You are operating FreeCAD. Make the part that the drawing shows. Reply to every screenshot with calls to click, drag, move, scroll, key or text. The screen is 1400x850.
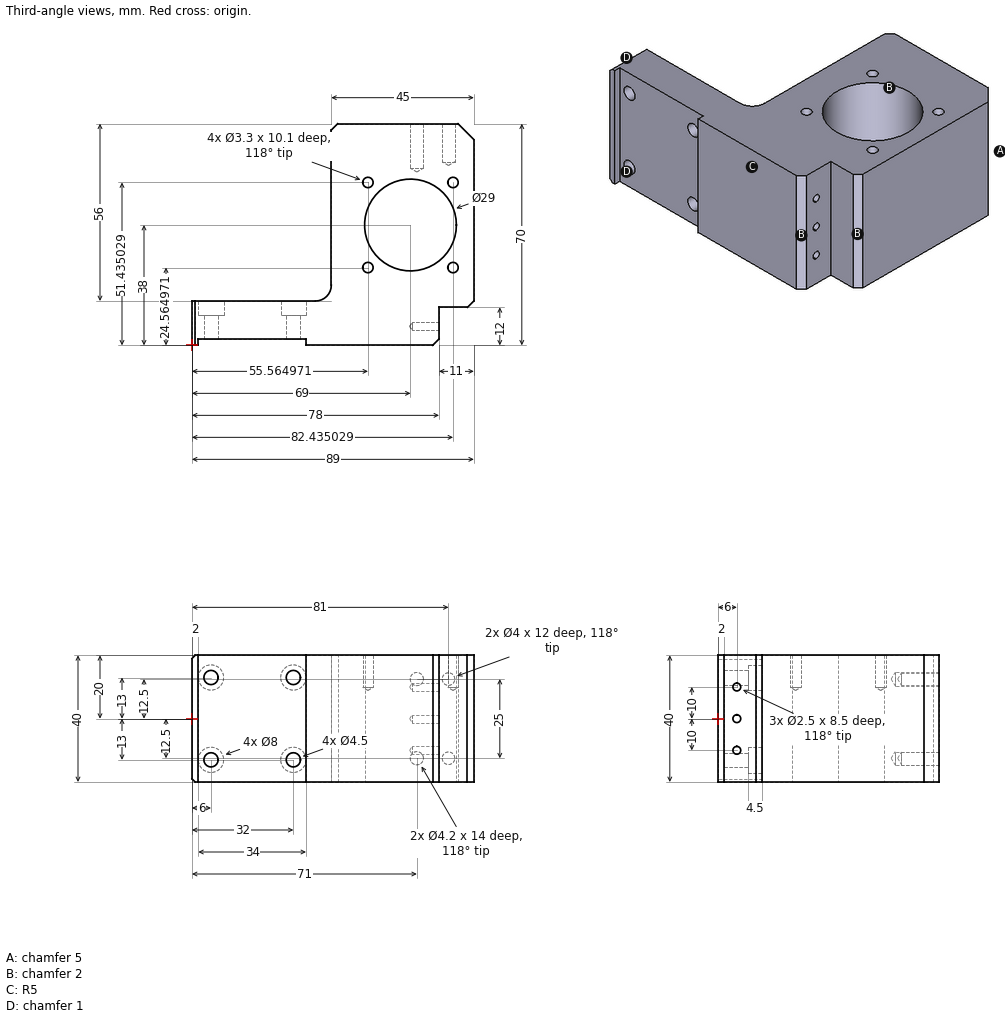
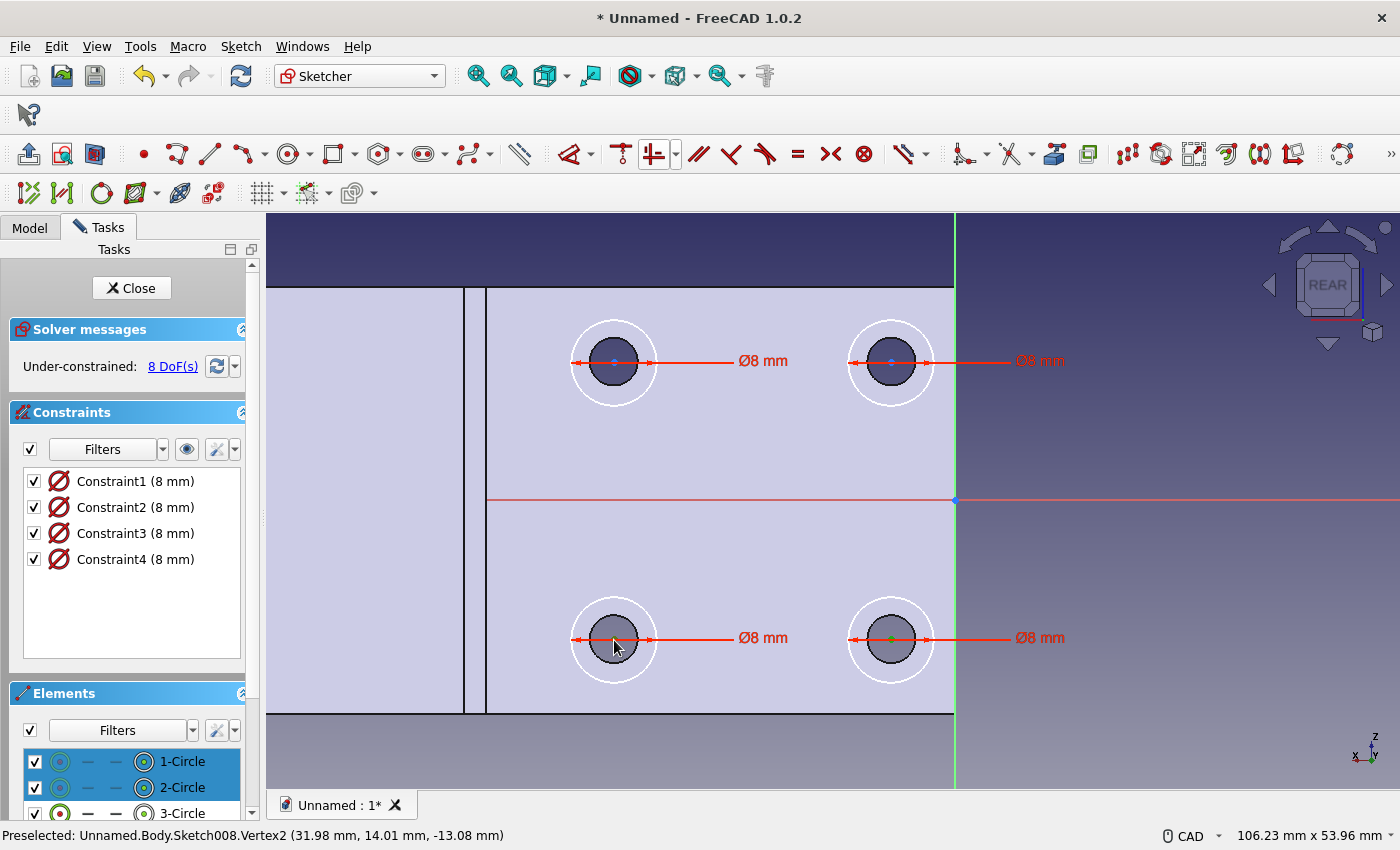
key(h)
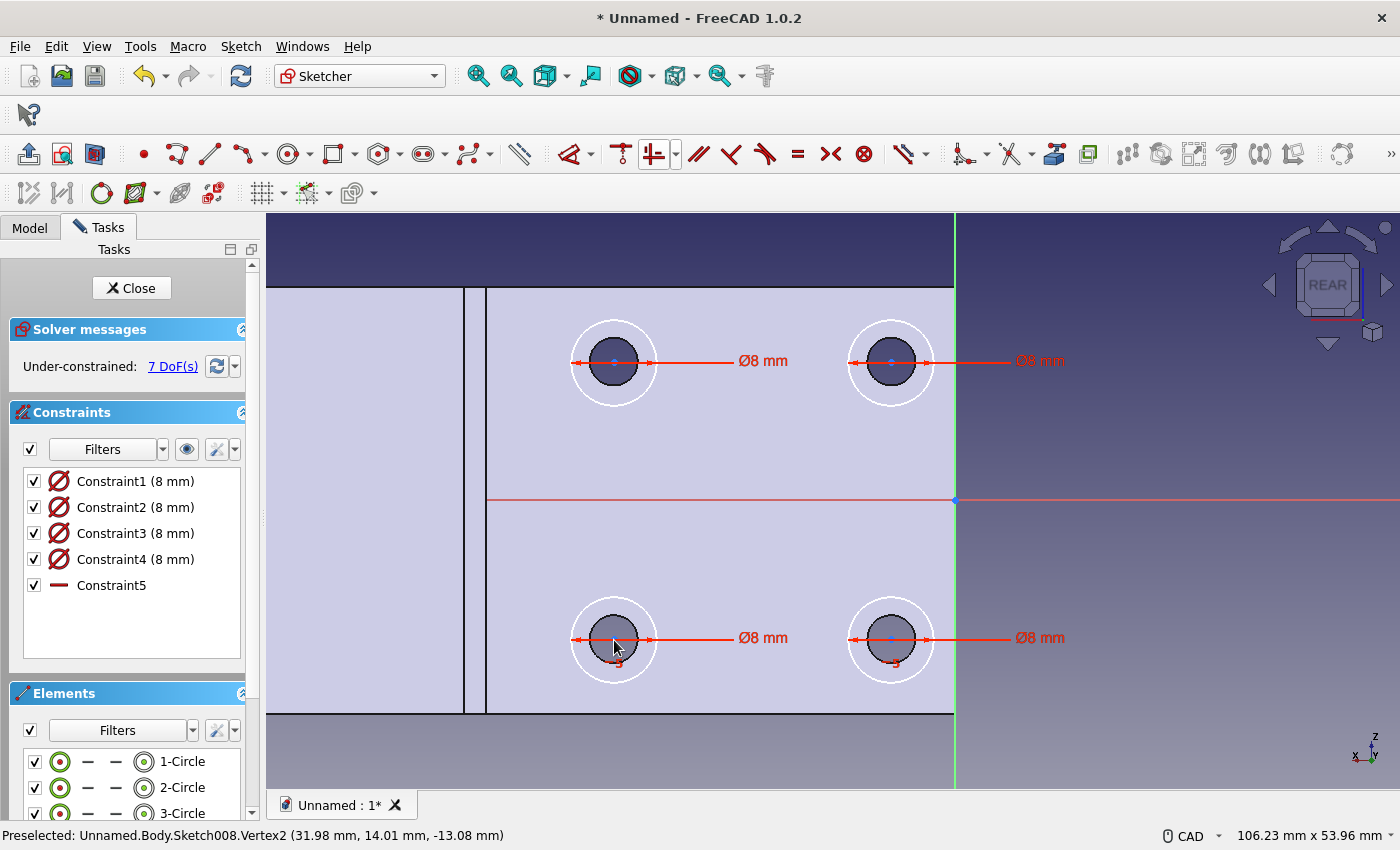
click(614, 640)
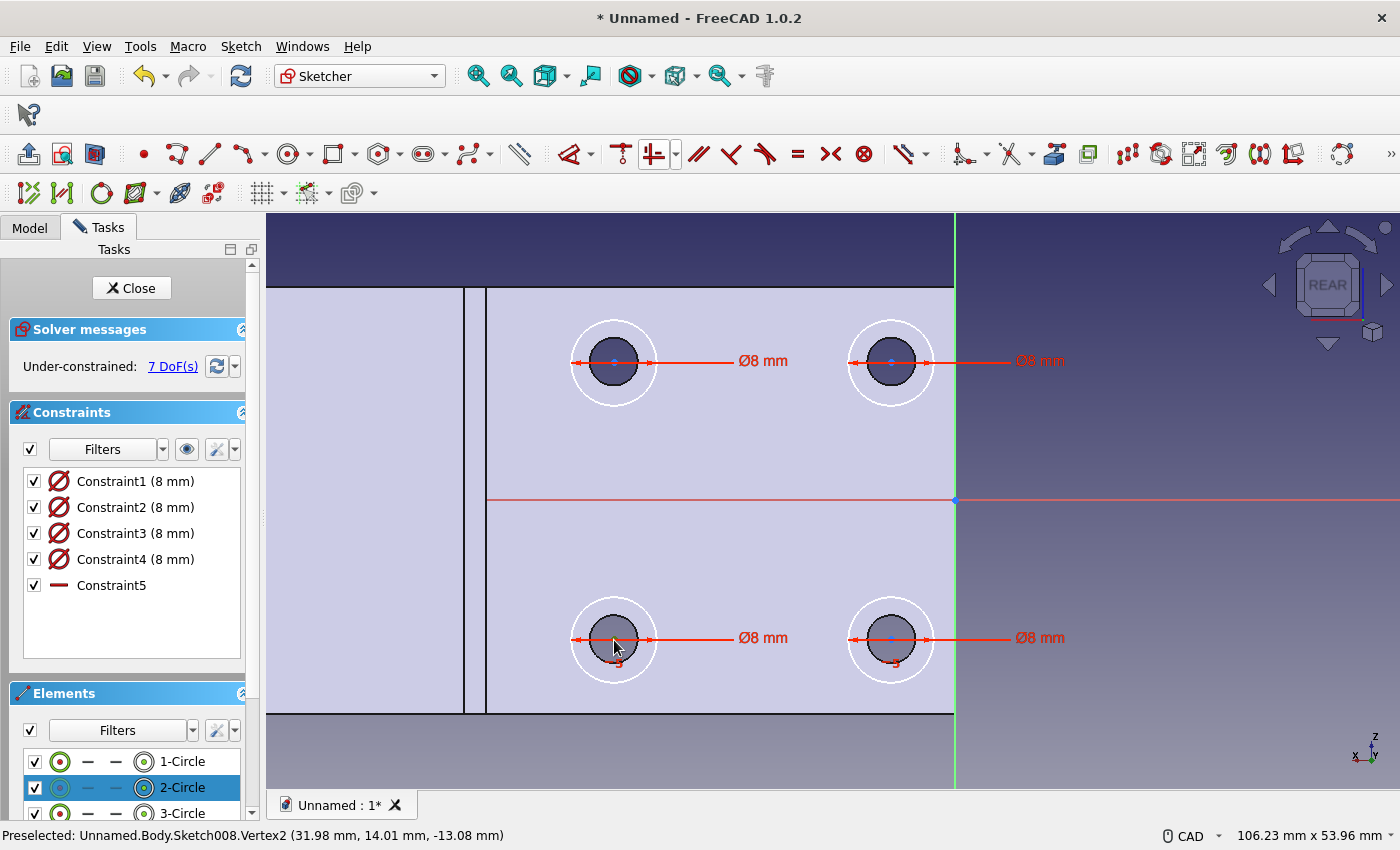
click(614, 363)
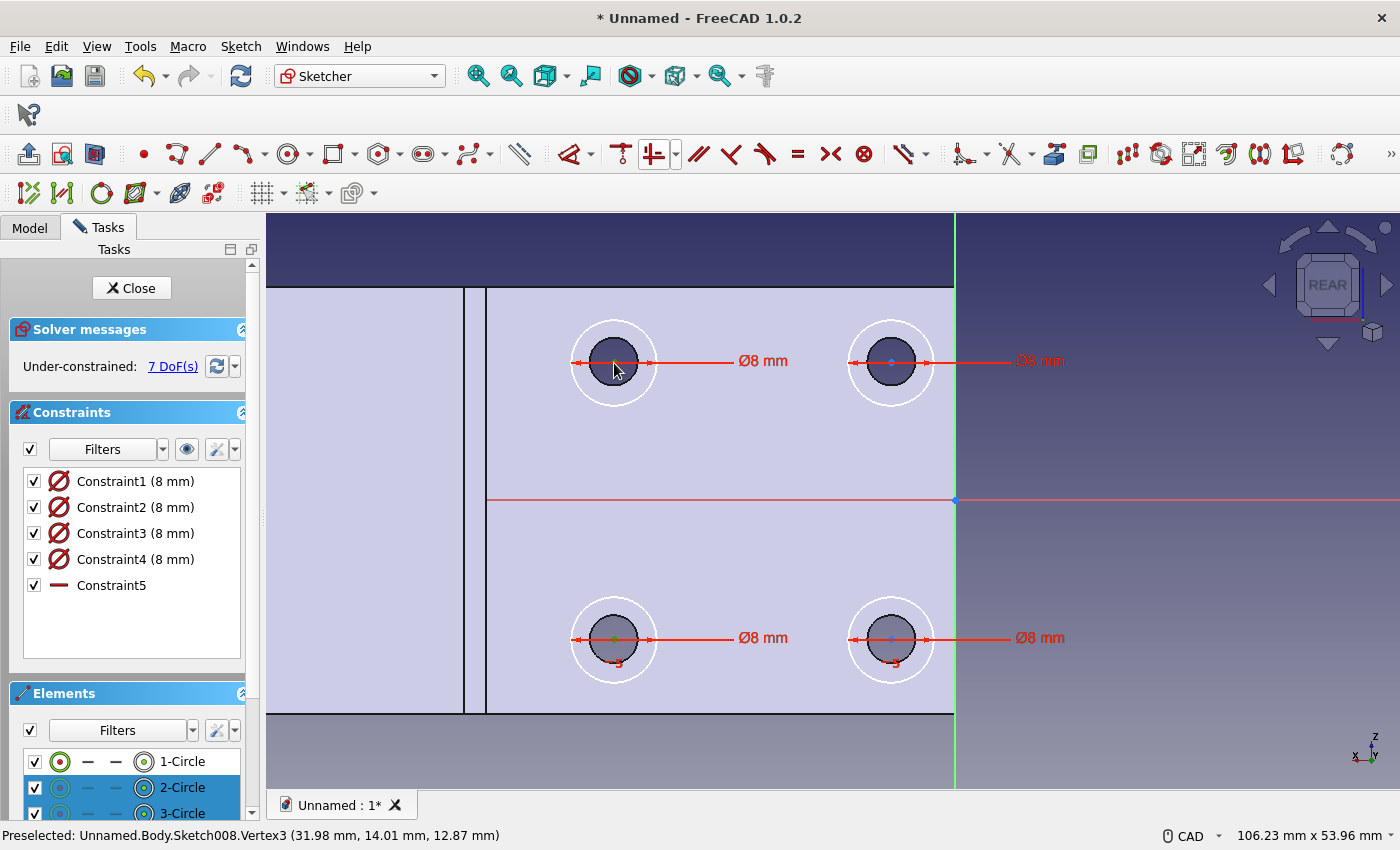
key(v)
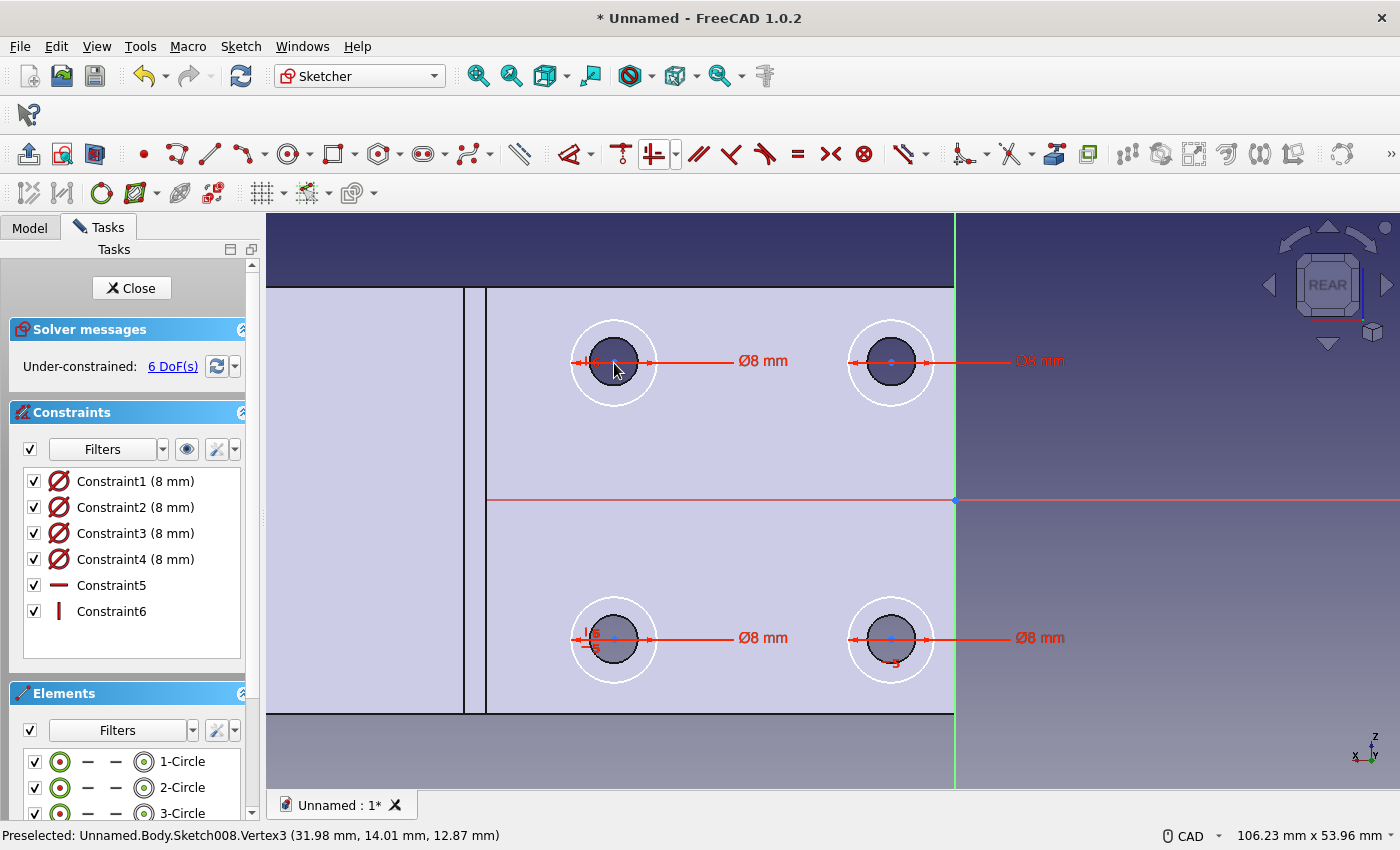
click(891, 640)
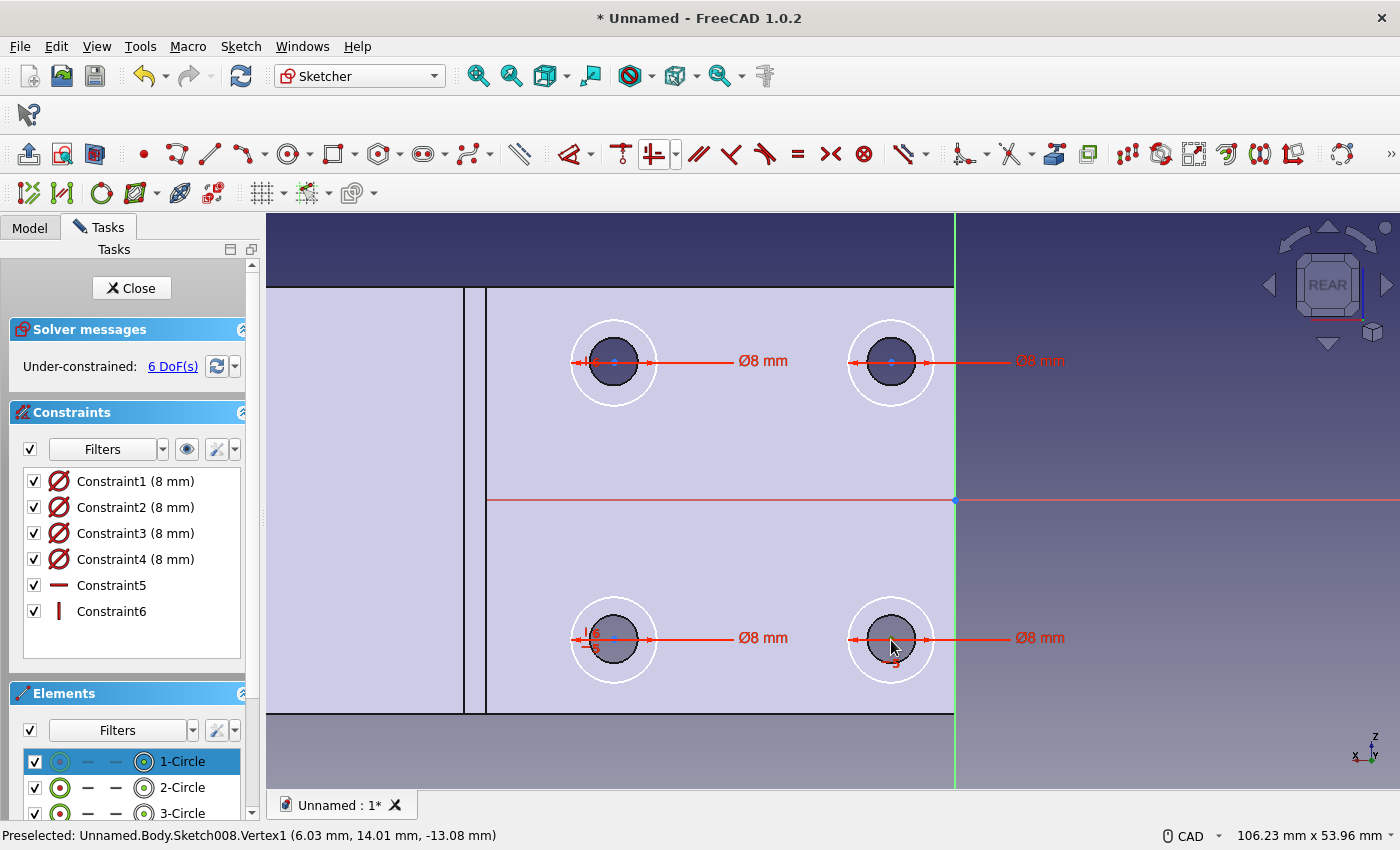
click(891, 363)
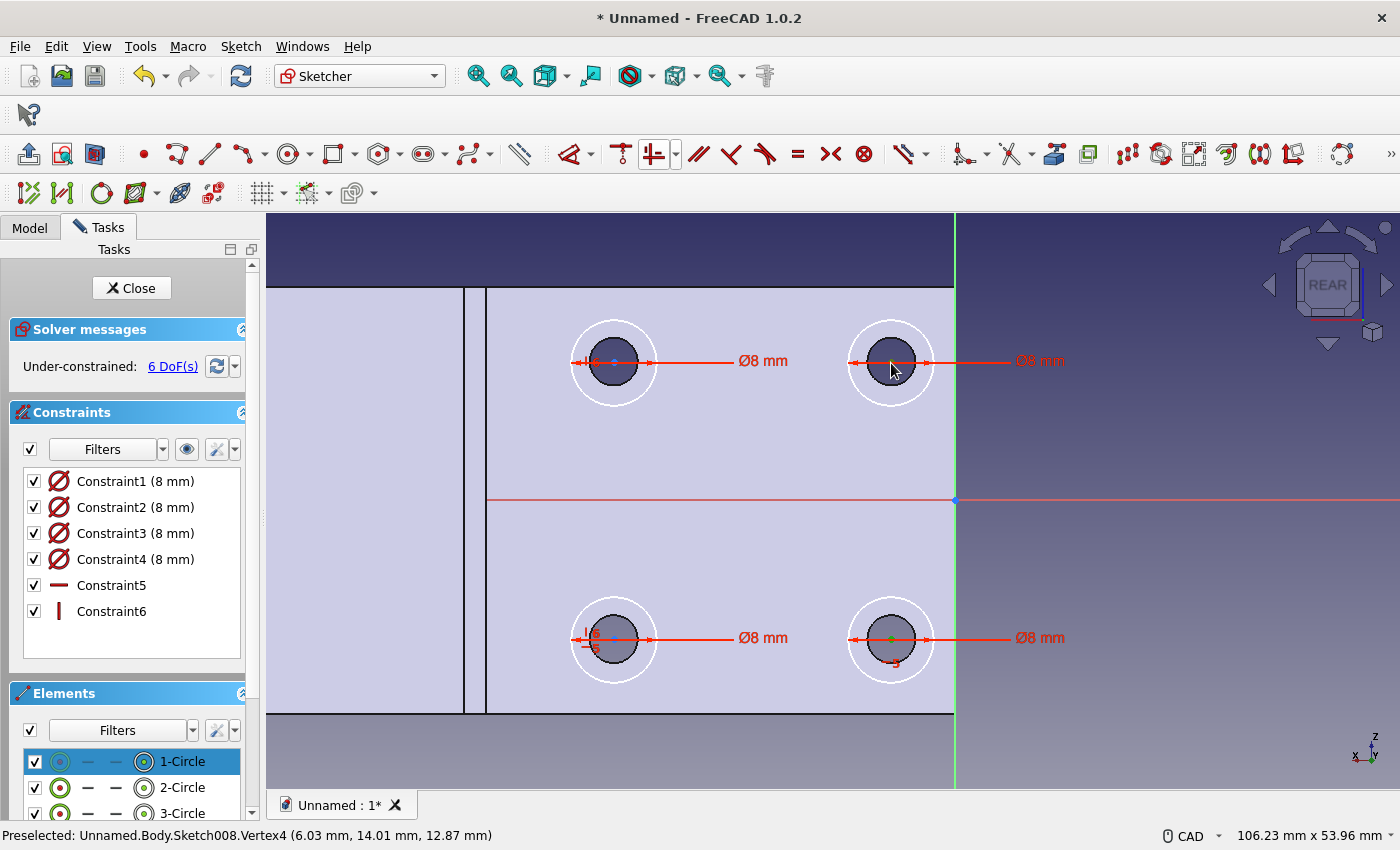
click(676, 154)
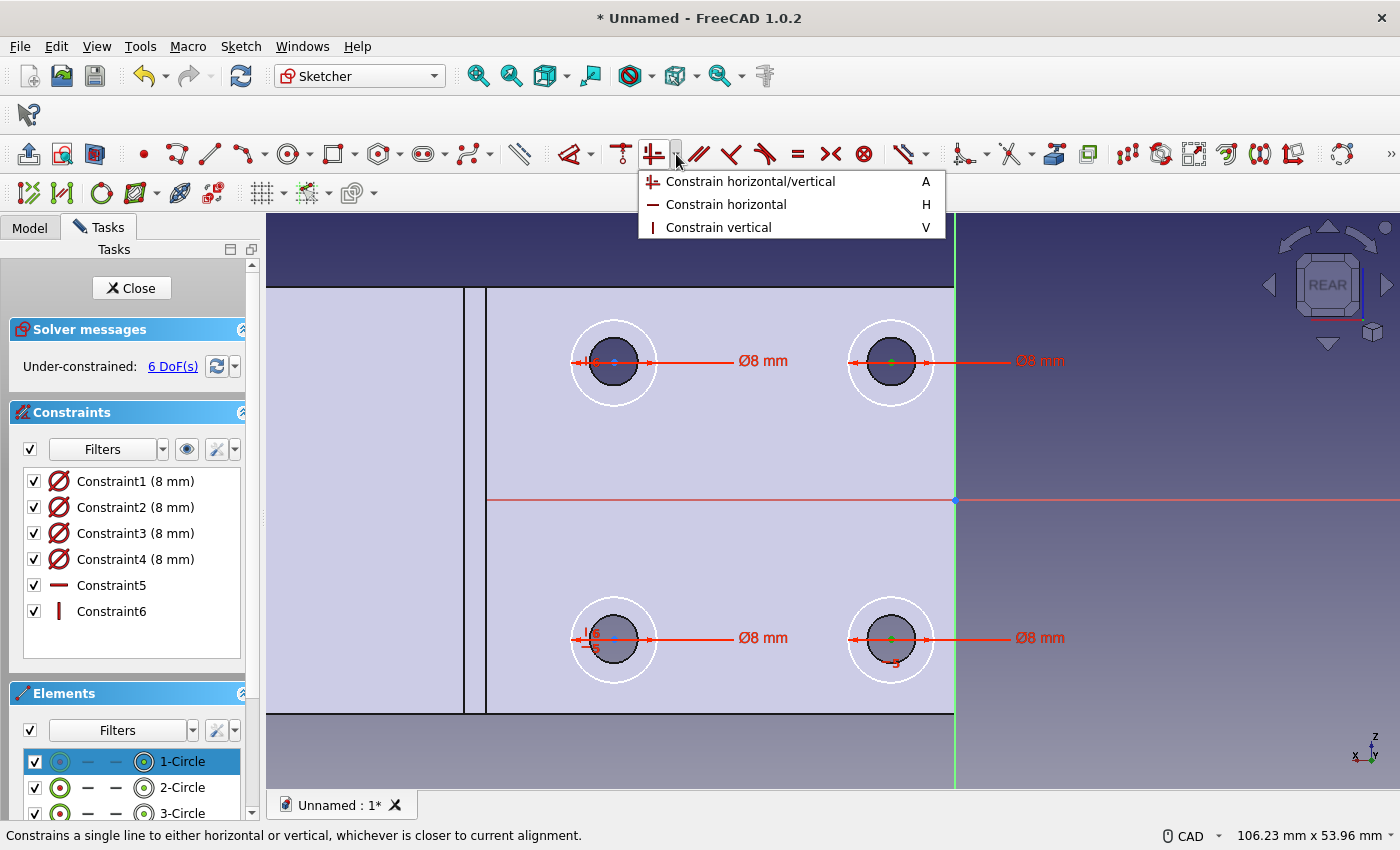
click(792, 228)